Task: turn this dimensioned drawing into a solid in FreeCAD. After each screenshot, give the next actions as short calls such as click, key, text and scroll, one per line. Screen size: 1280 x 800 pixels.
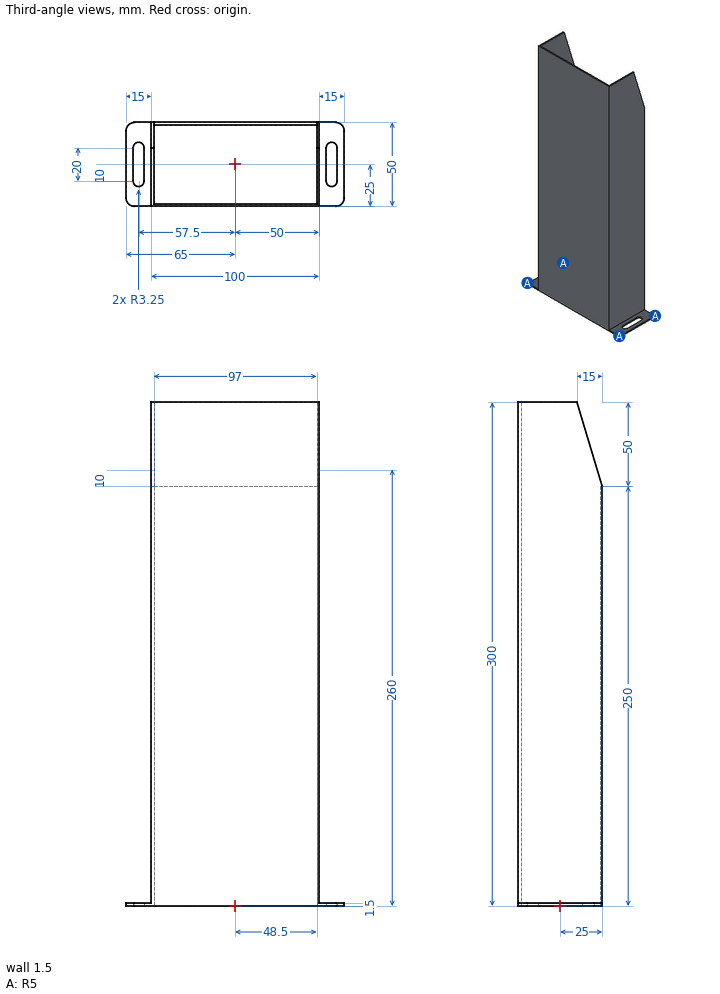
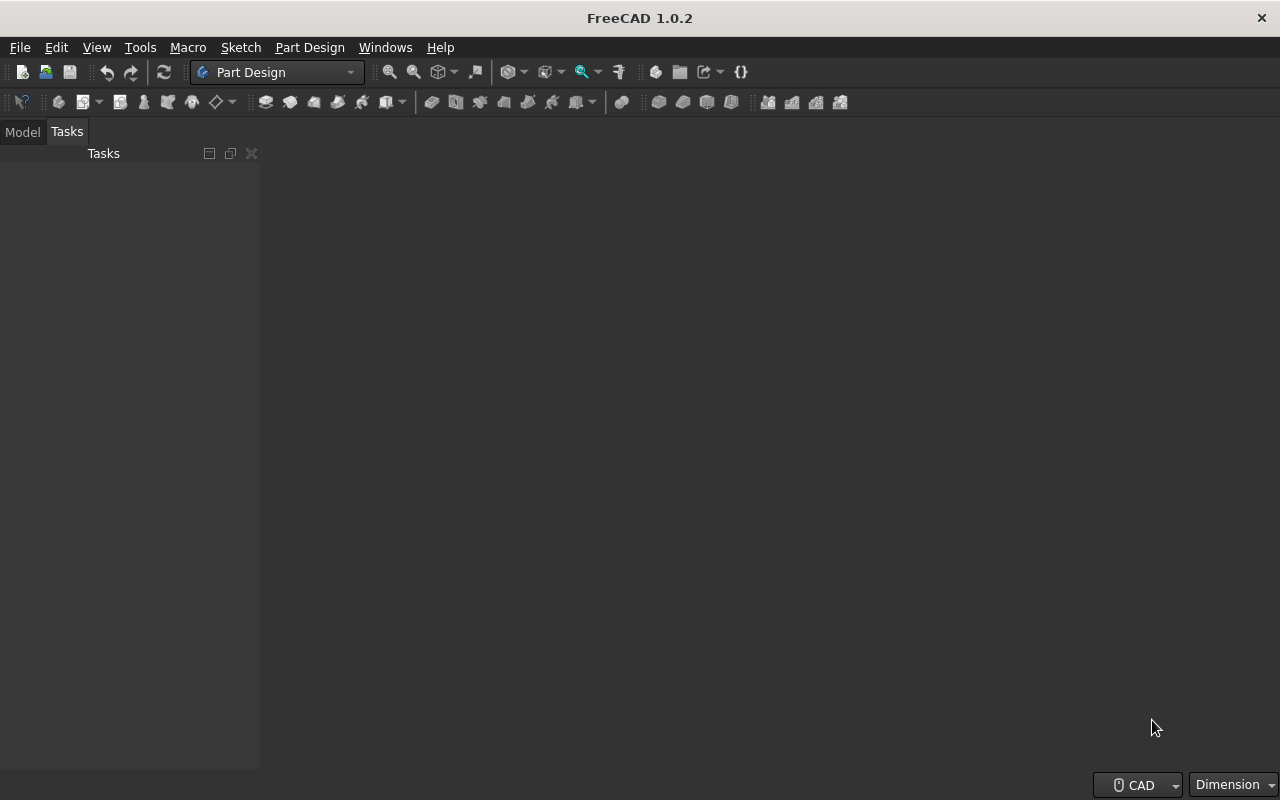
click(22, 72)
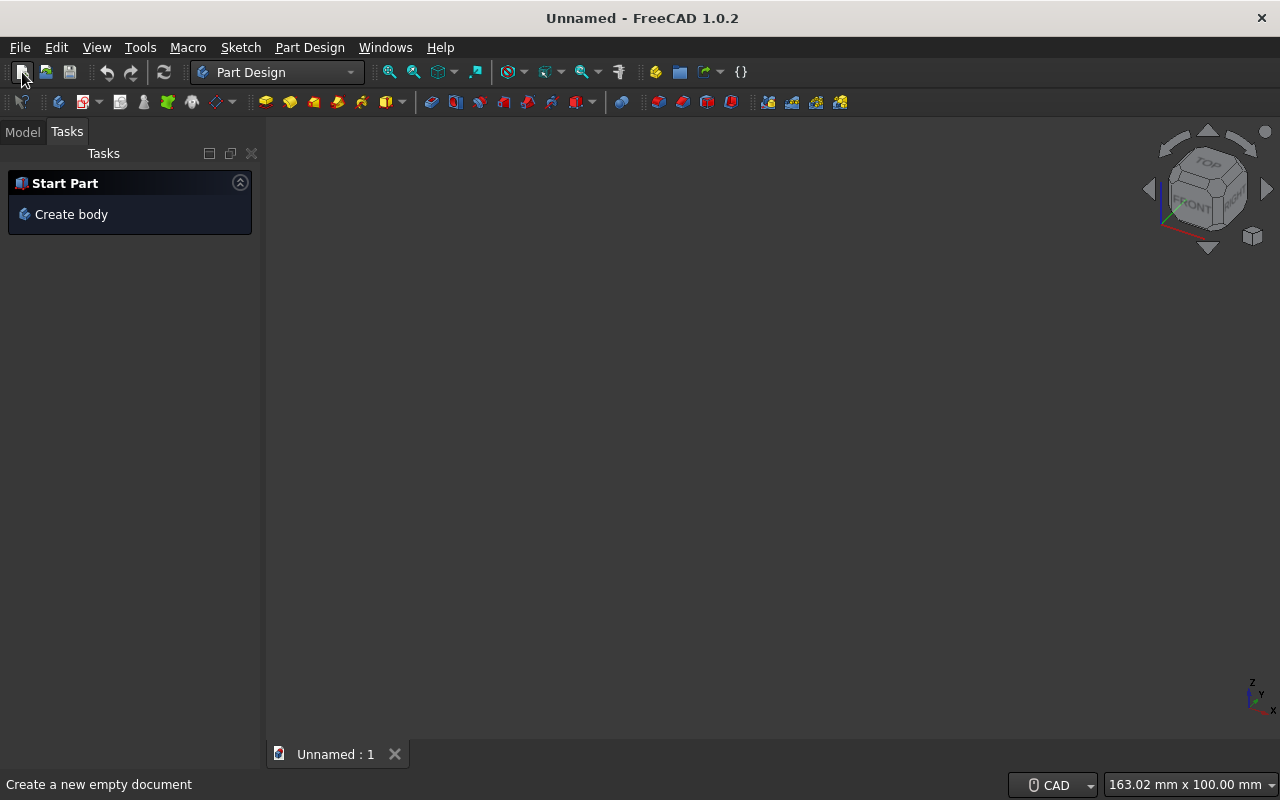
click(84, 102)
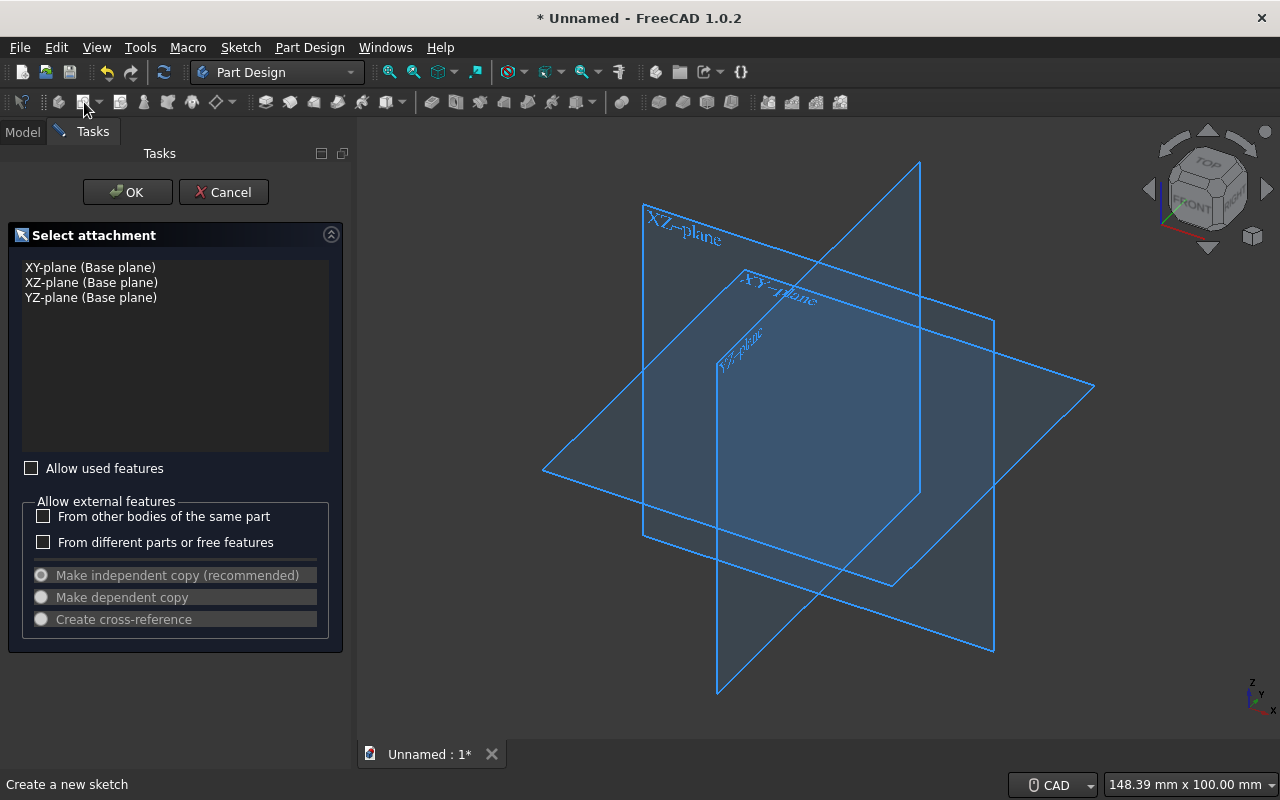
click(82, 268)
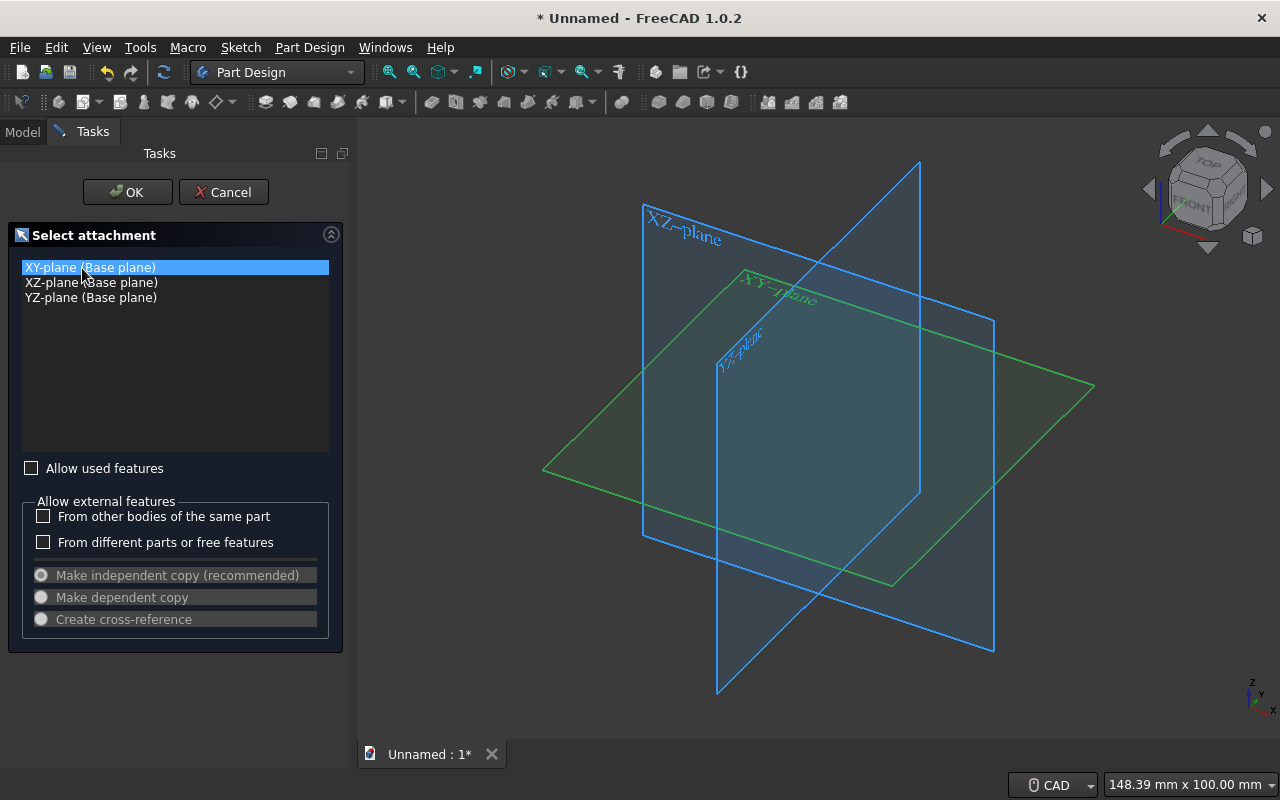
click(128, 192)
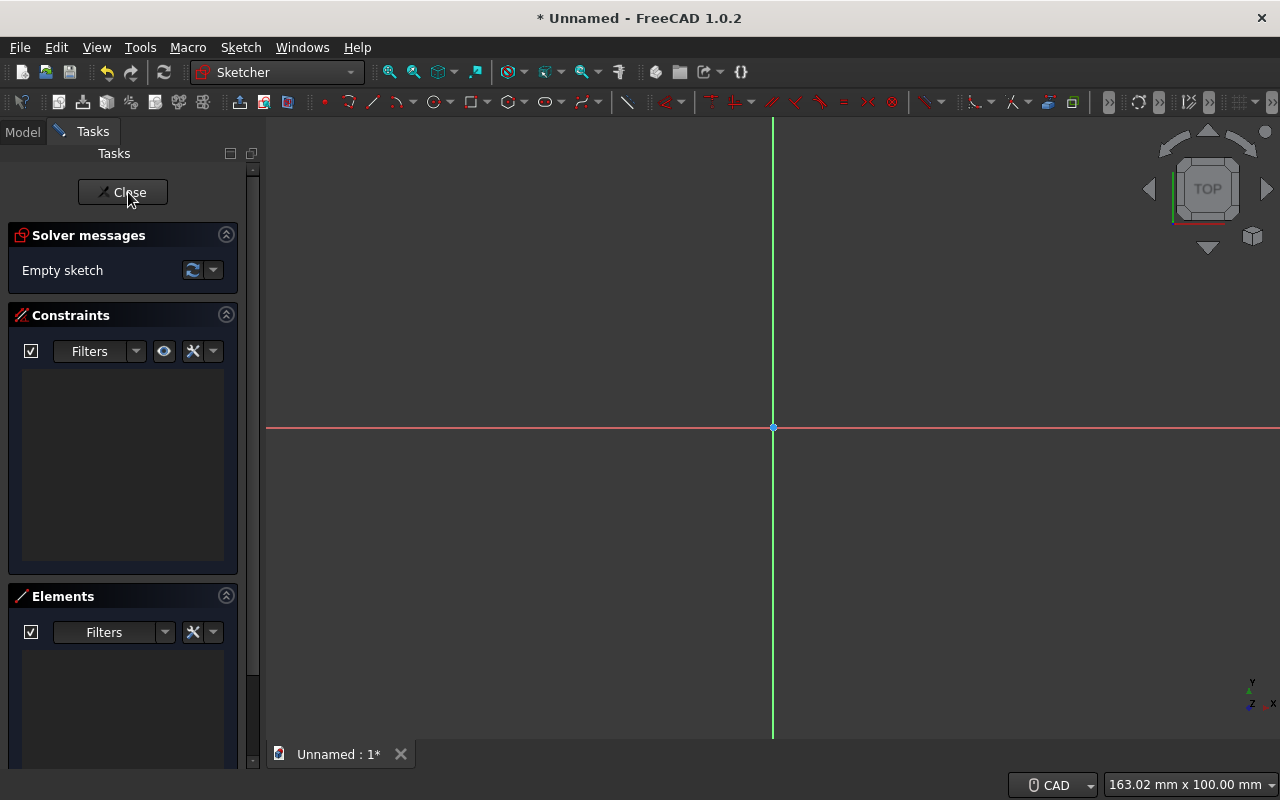
click(490, 102)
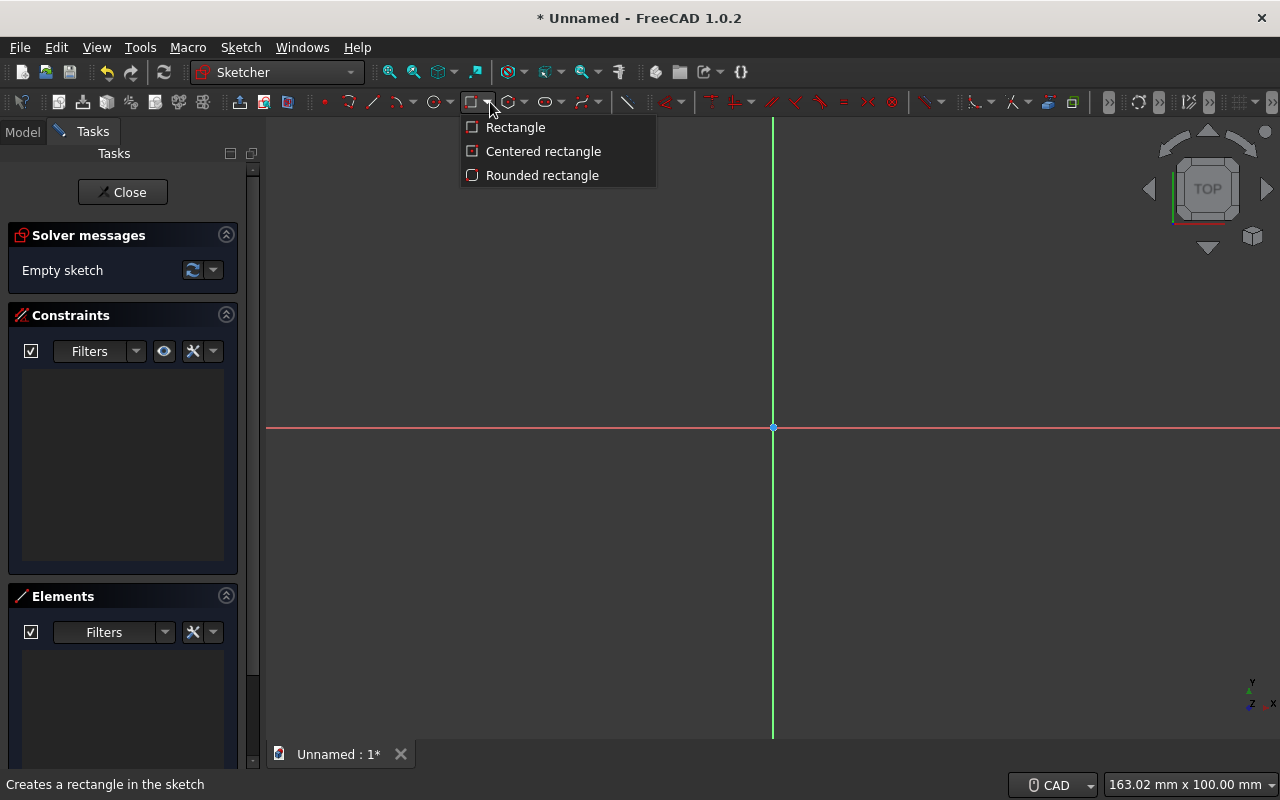
click(558, 151)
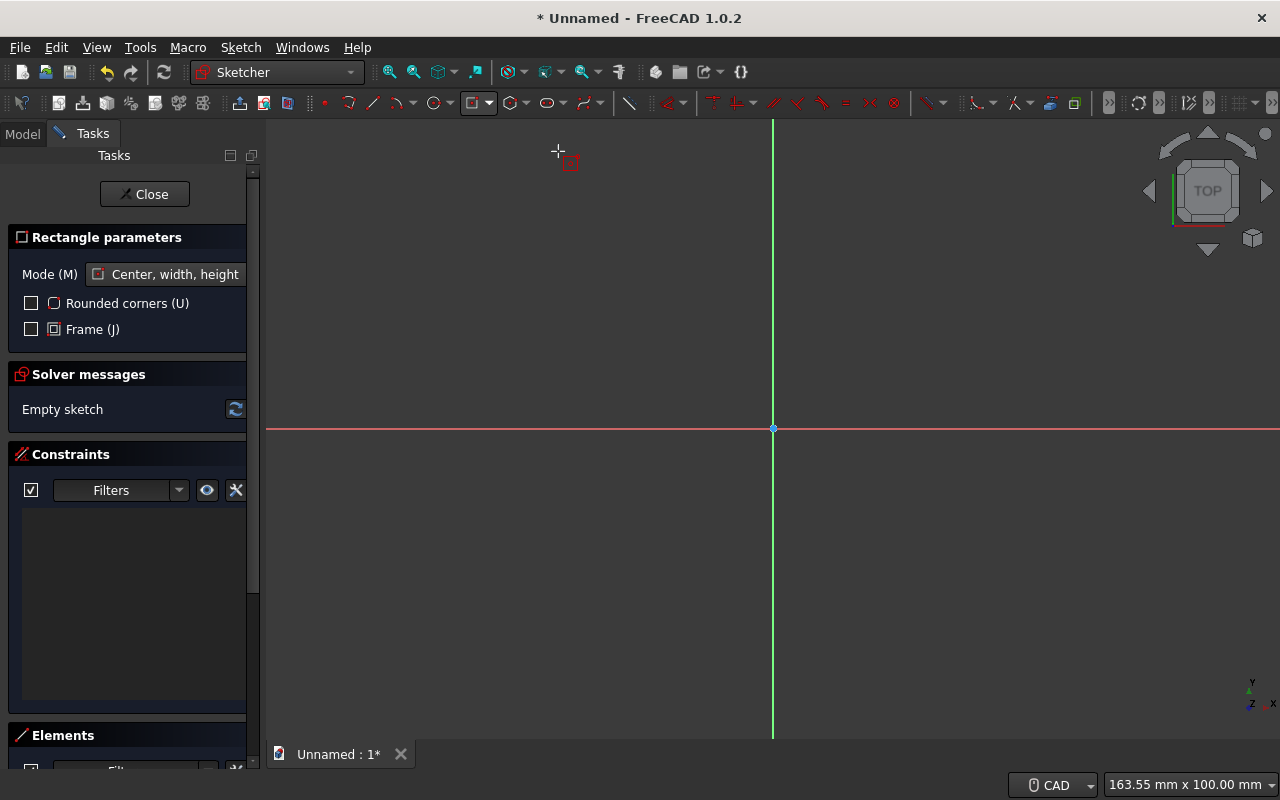
click(773, 429)
move(1083, 274)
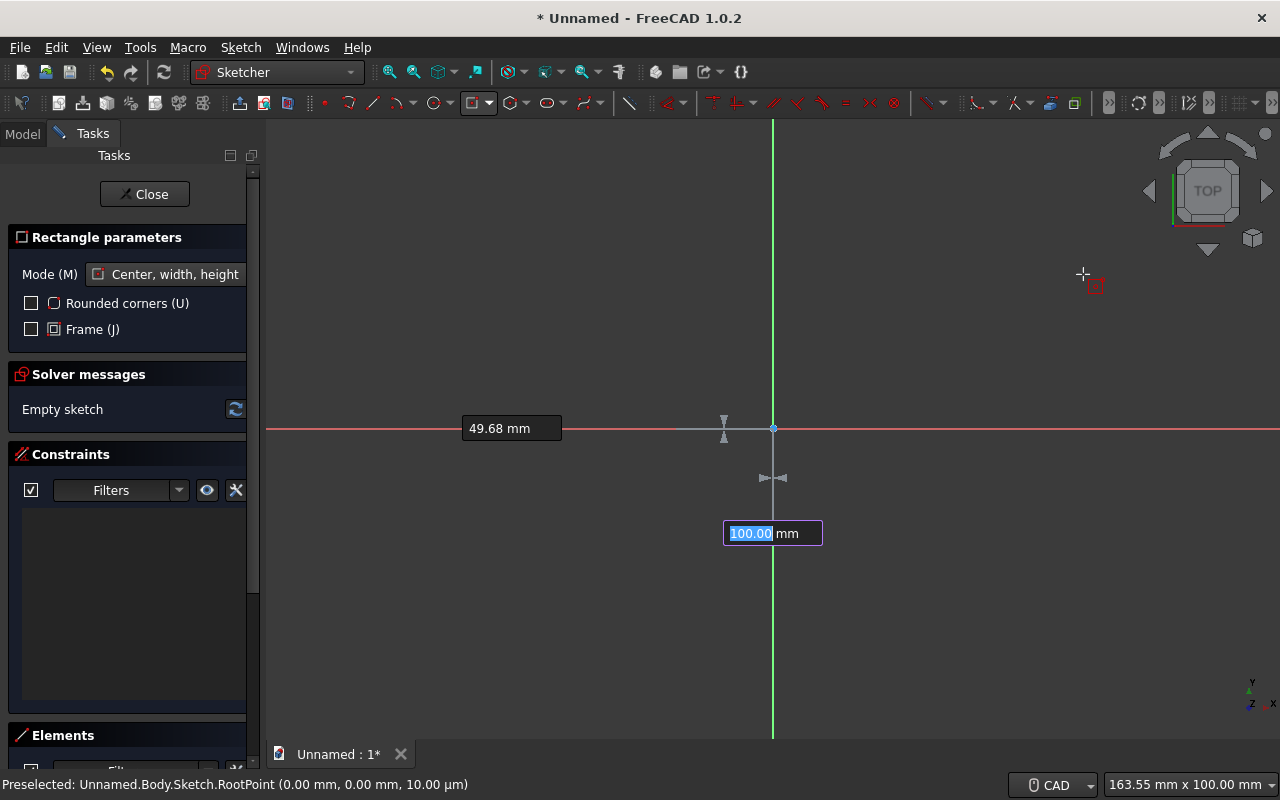
text(100)
key(Tab)
text(50)
key(Return)
key(Escape)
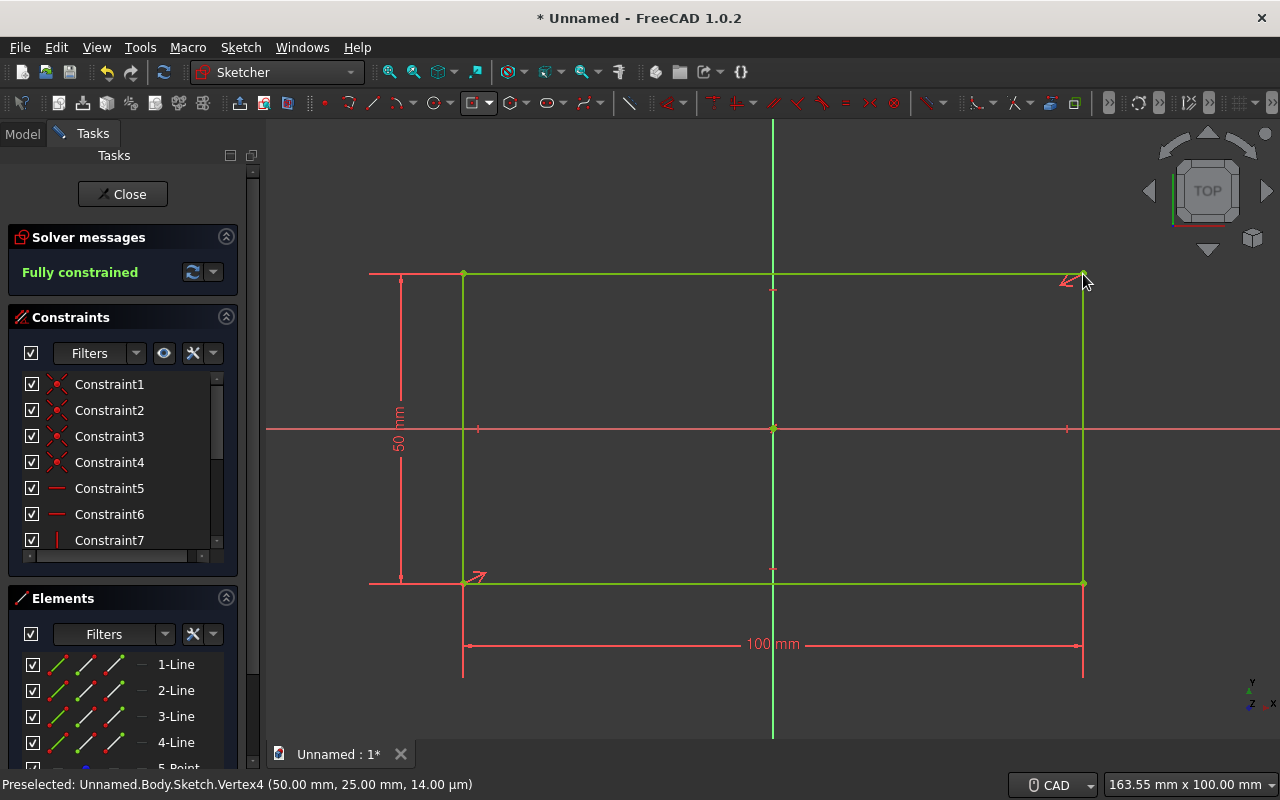
click(123, 194)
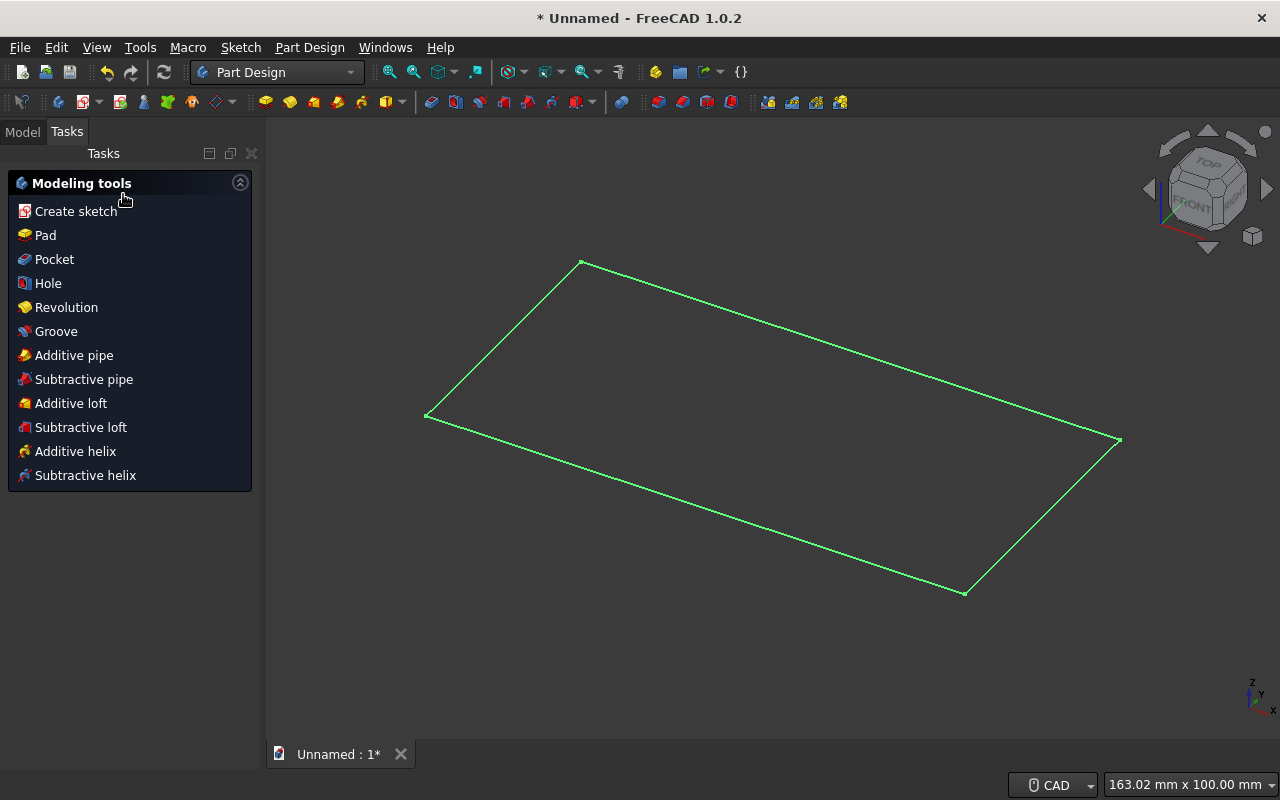
click(266, 102)